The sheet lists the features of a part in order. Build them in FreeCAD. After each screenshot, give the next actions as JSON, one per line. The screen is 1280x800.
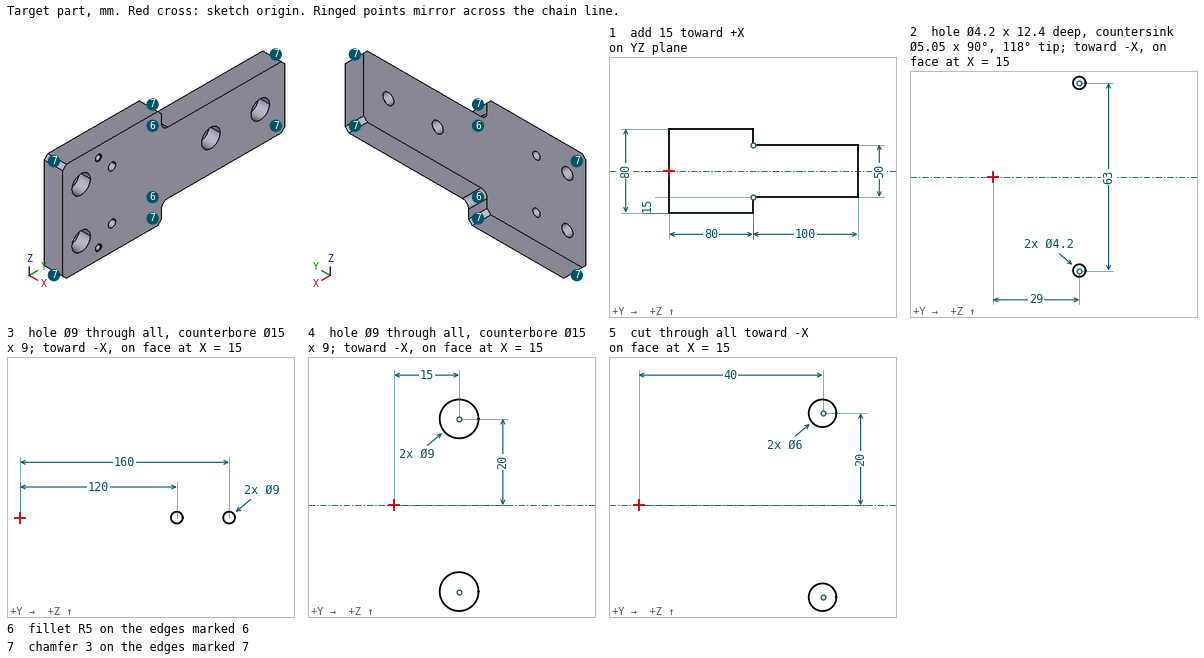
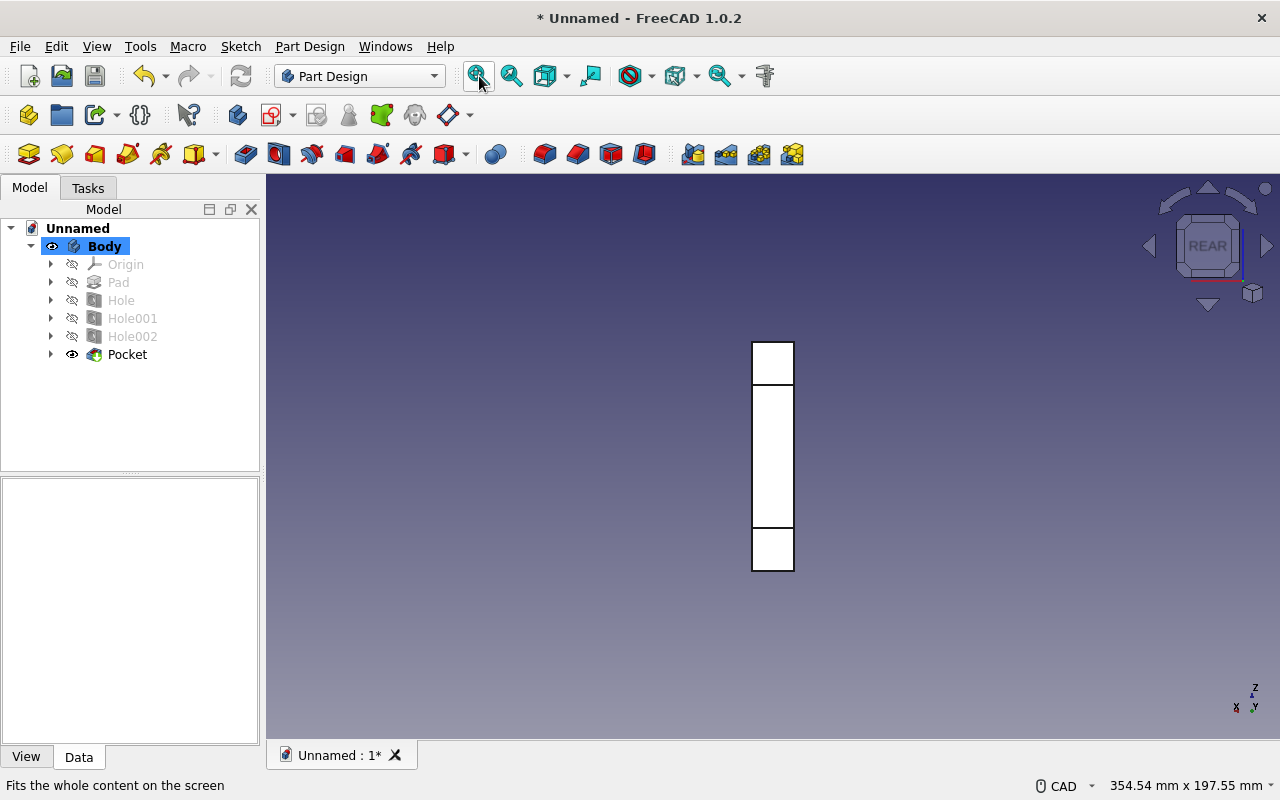
{"action": "key", "text": "6"}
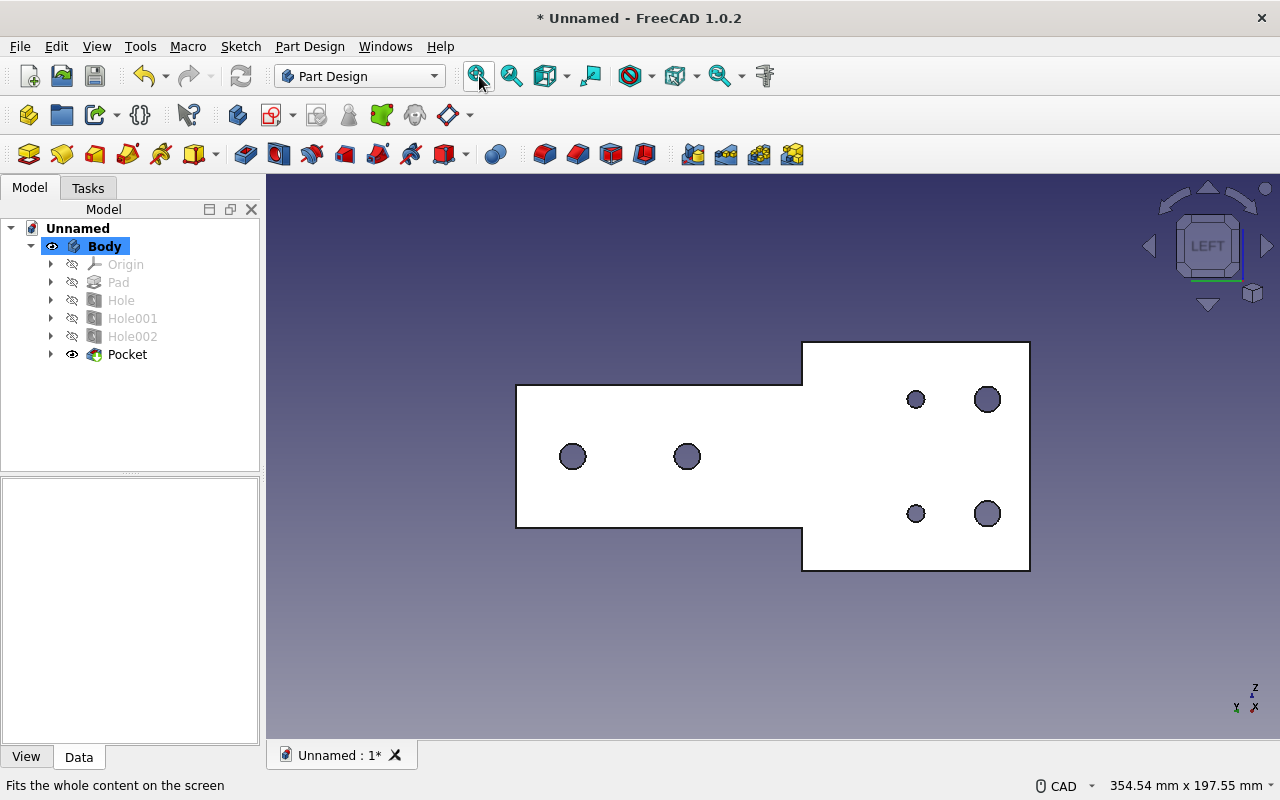
{"action": "key", "text": "v 3"}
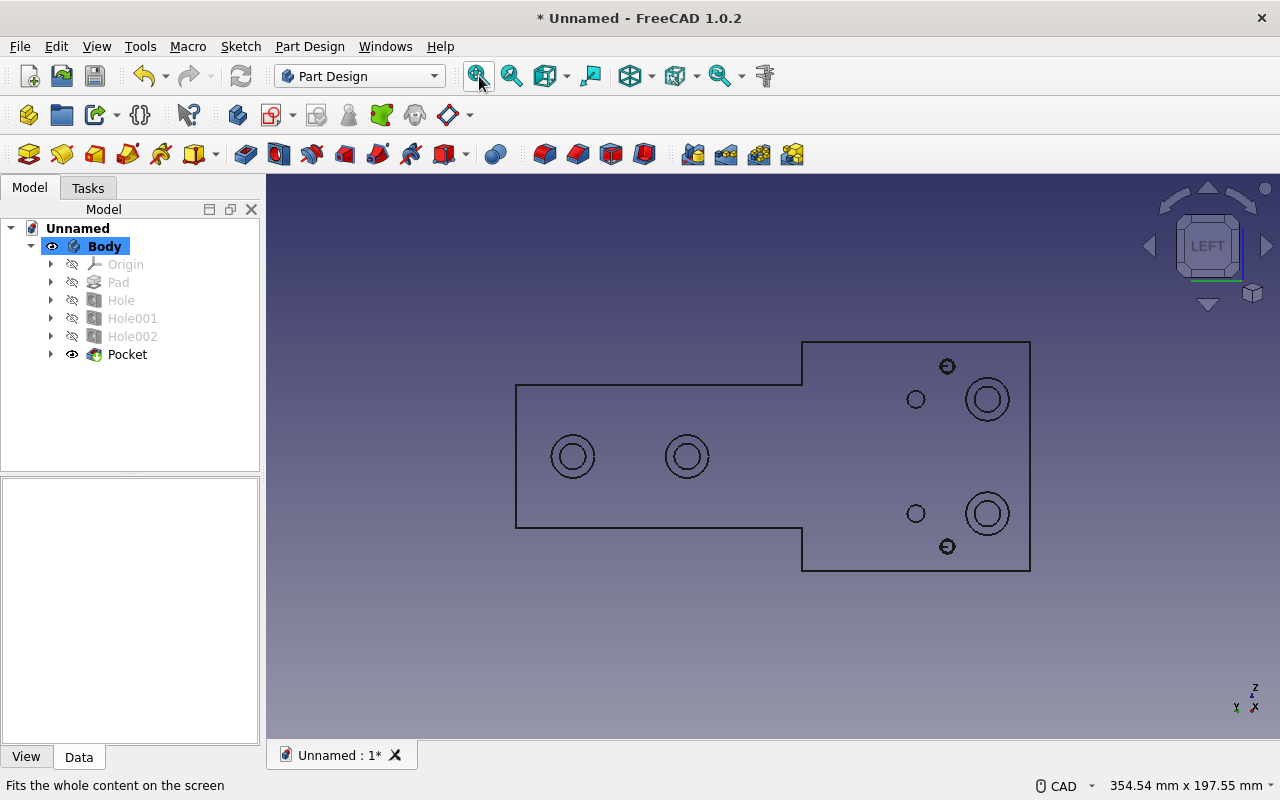
{"action": "key", "text": "0"}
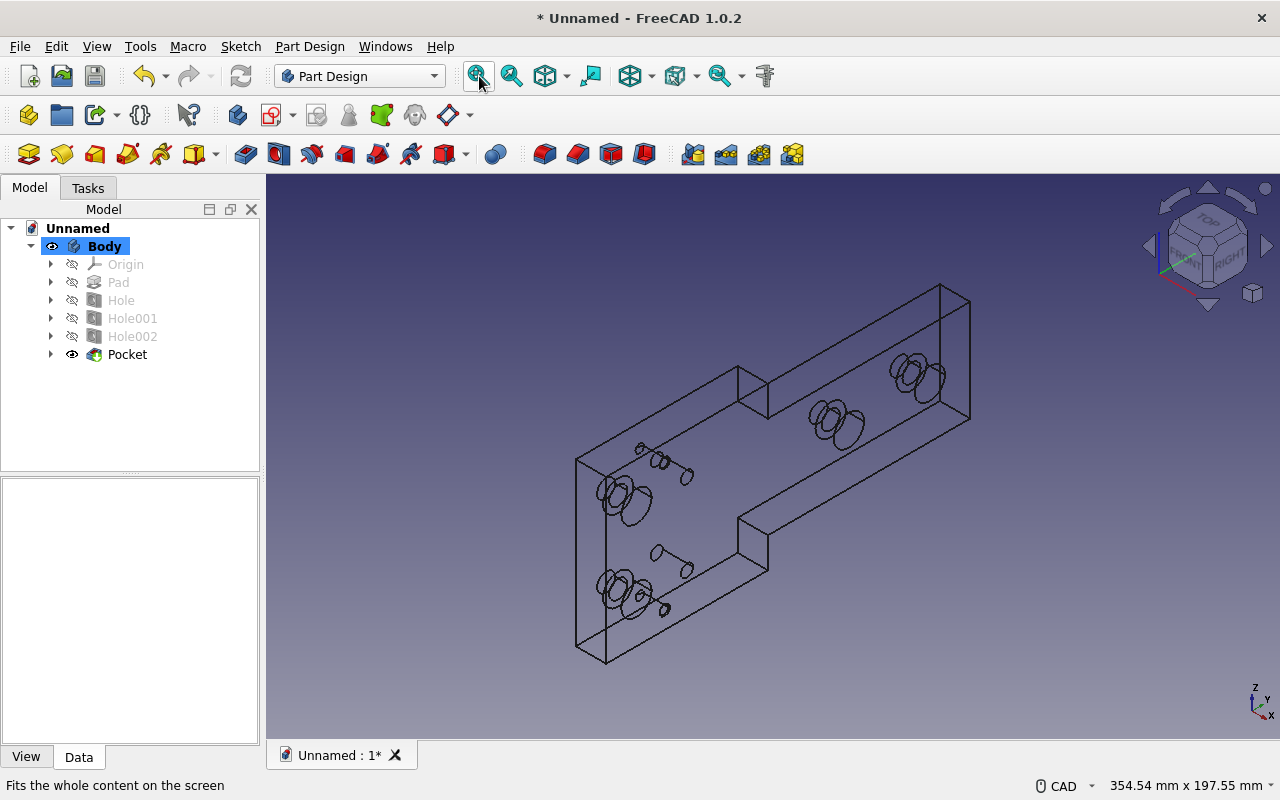
{"action": "left_click", "coordinate": [753, 409]}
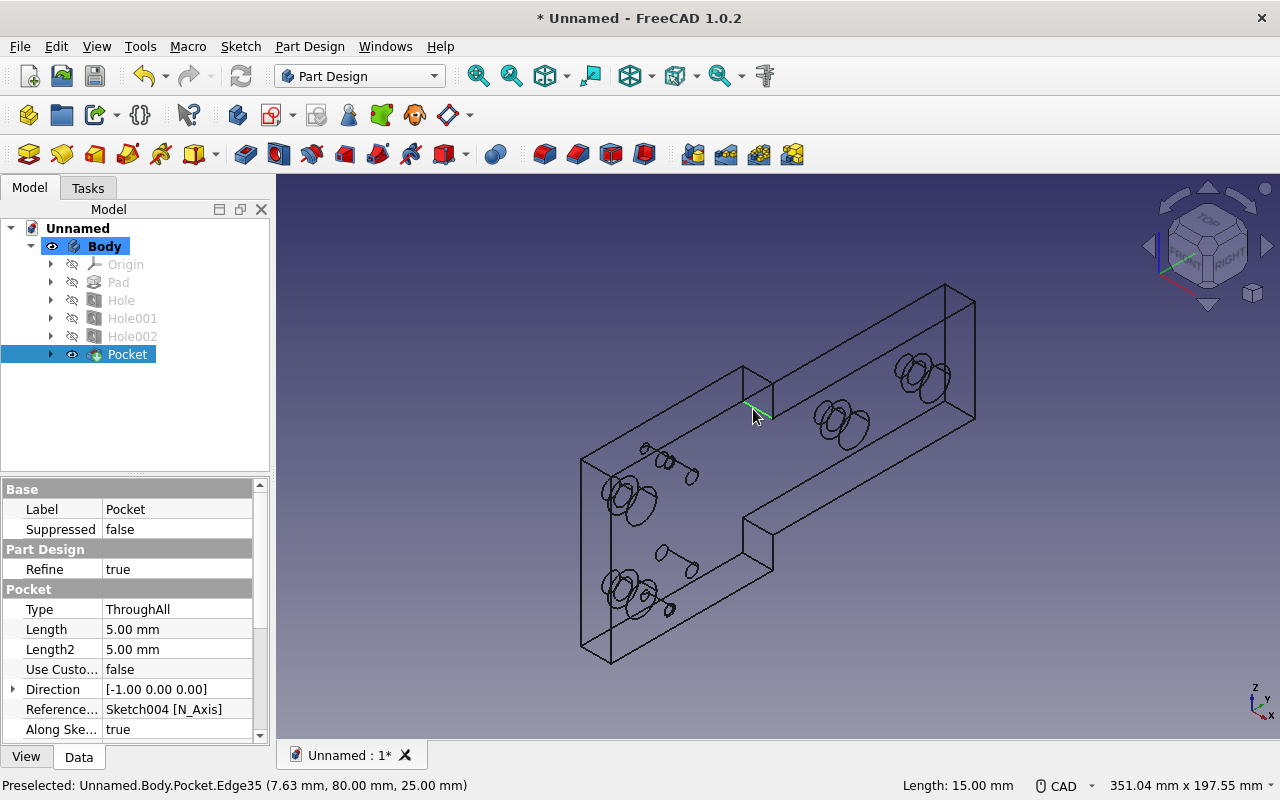
{"action": "left_click", "coordinate": [758, 526], "text": "ctrl"}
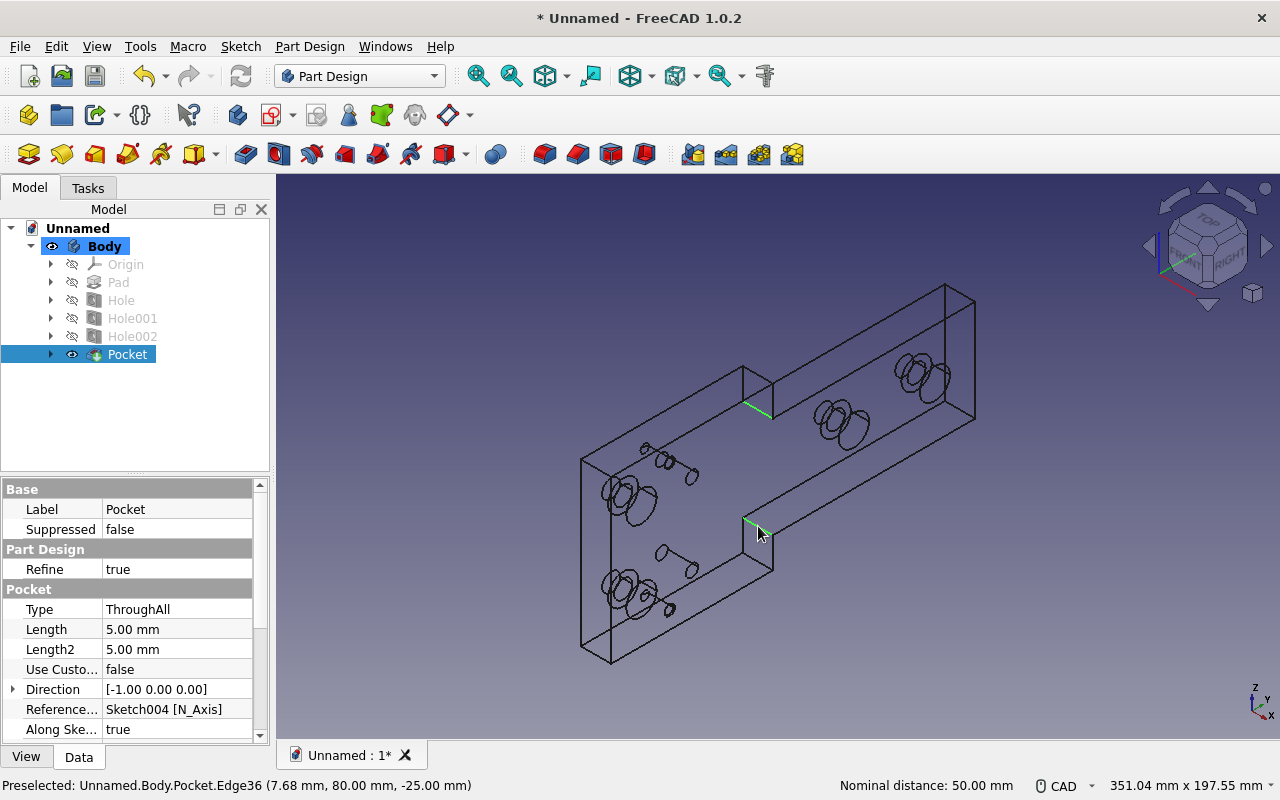
{"action": "key", "text": "v 1"}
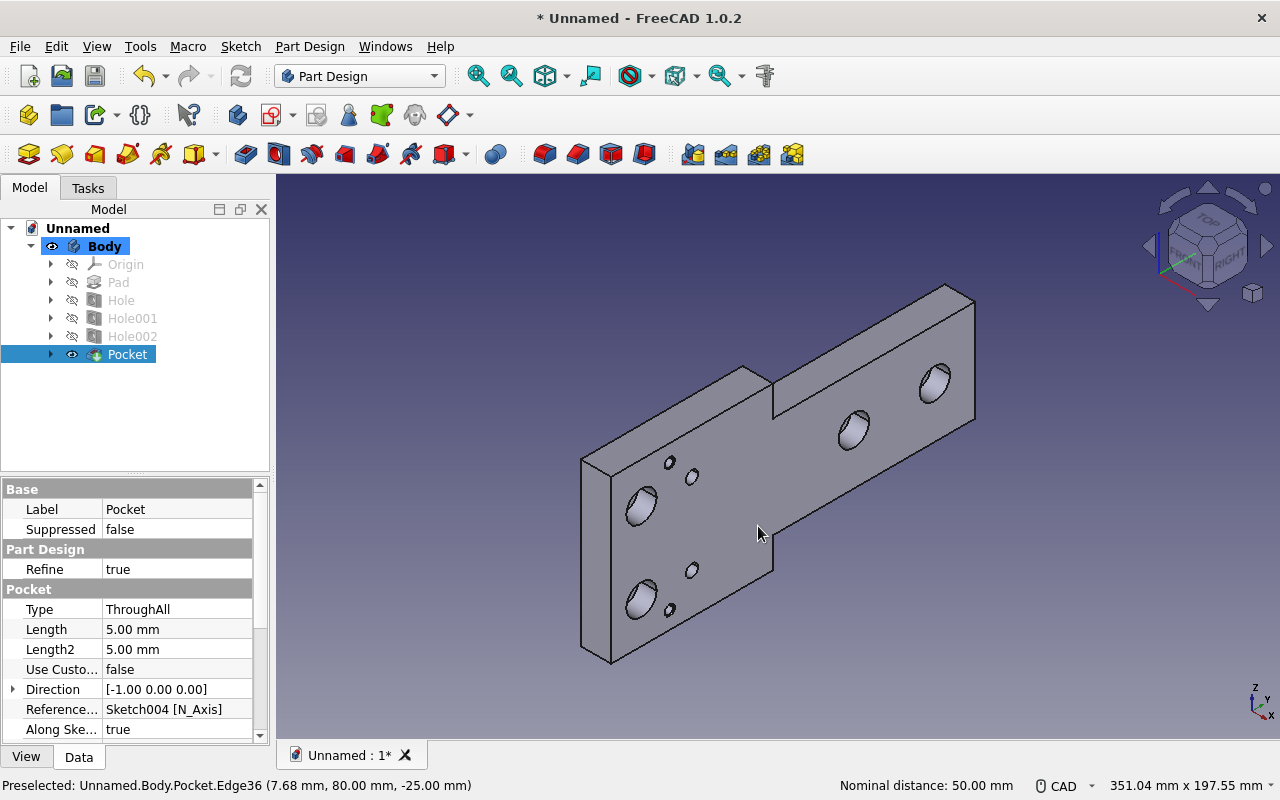
{"action": "left_click", "coordinate": [545, 154]}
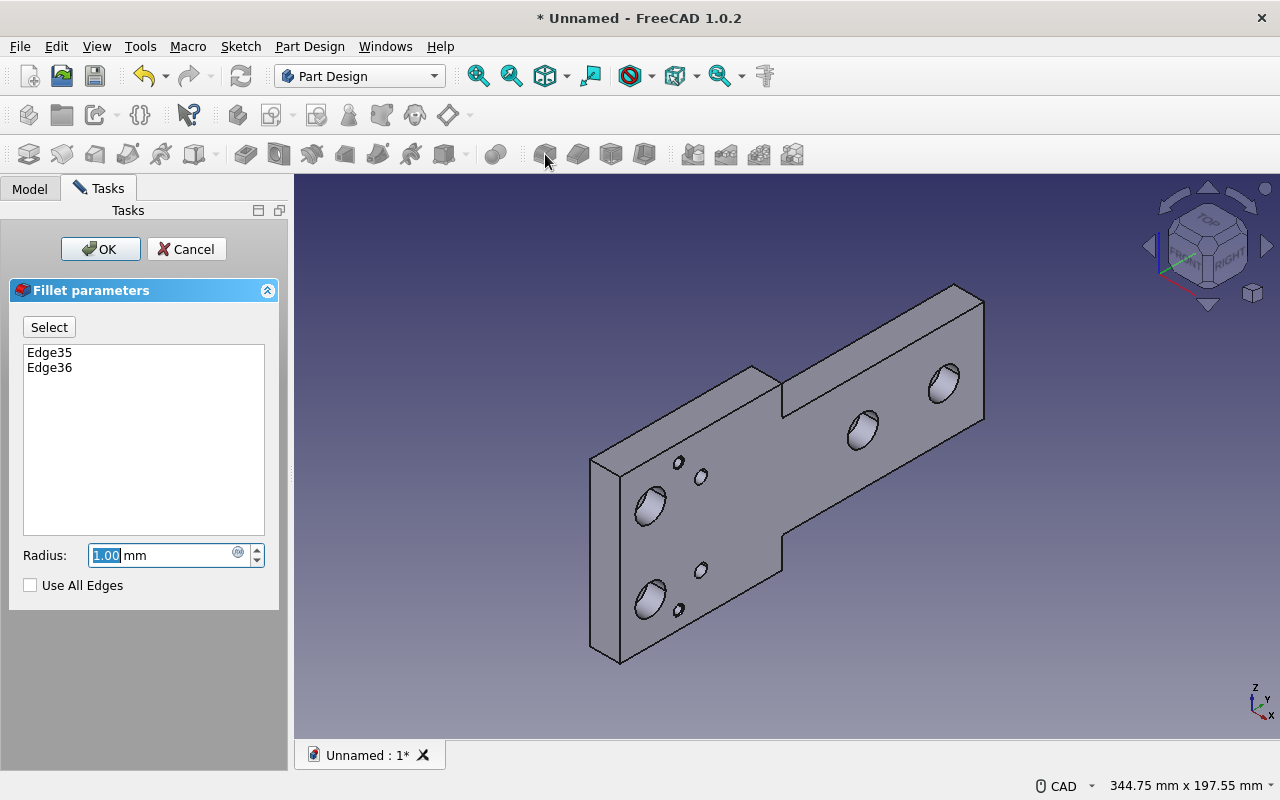
{"action": "type", "text": "5"}
{"action": "key", "text": "Tab"}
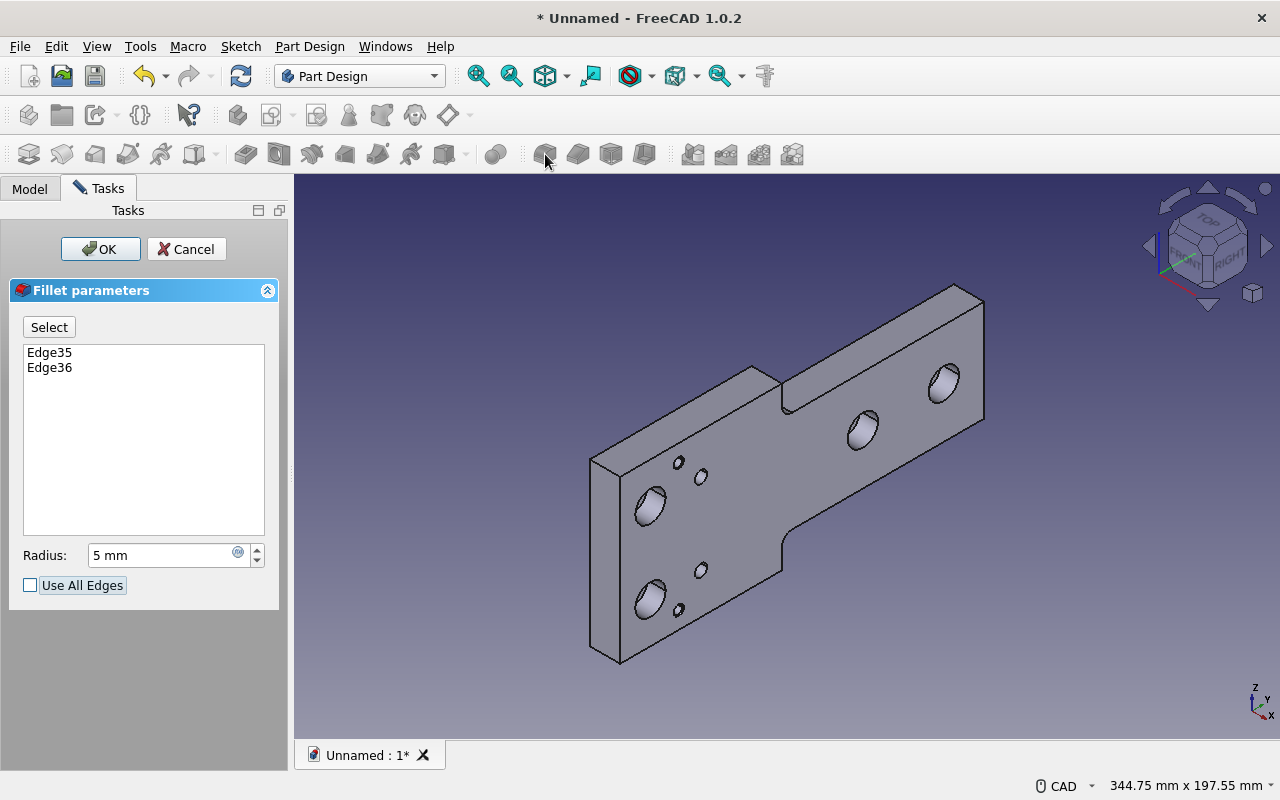
{"action": "left_click", "coordinate": [101, 249]}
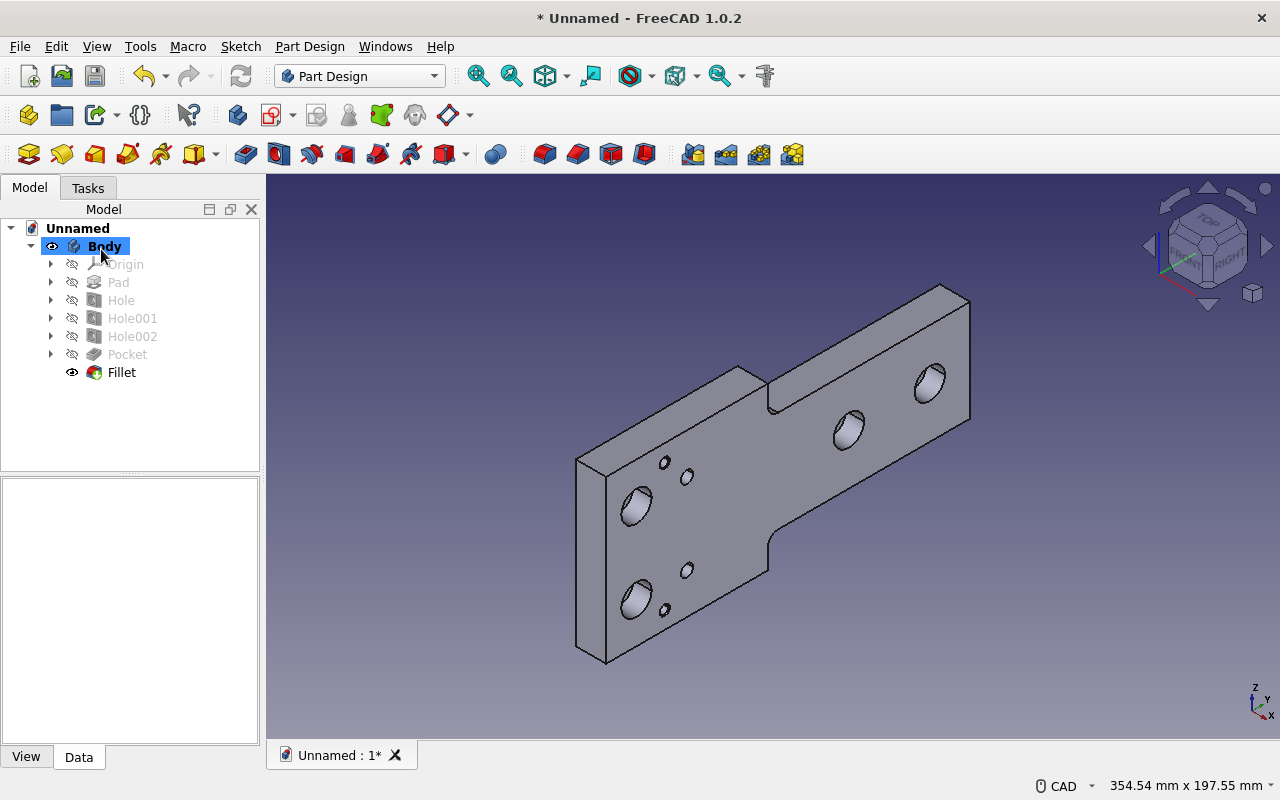
{"action": "left_click", "coordinate": [591, 467]}